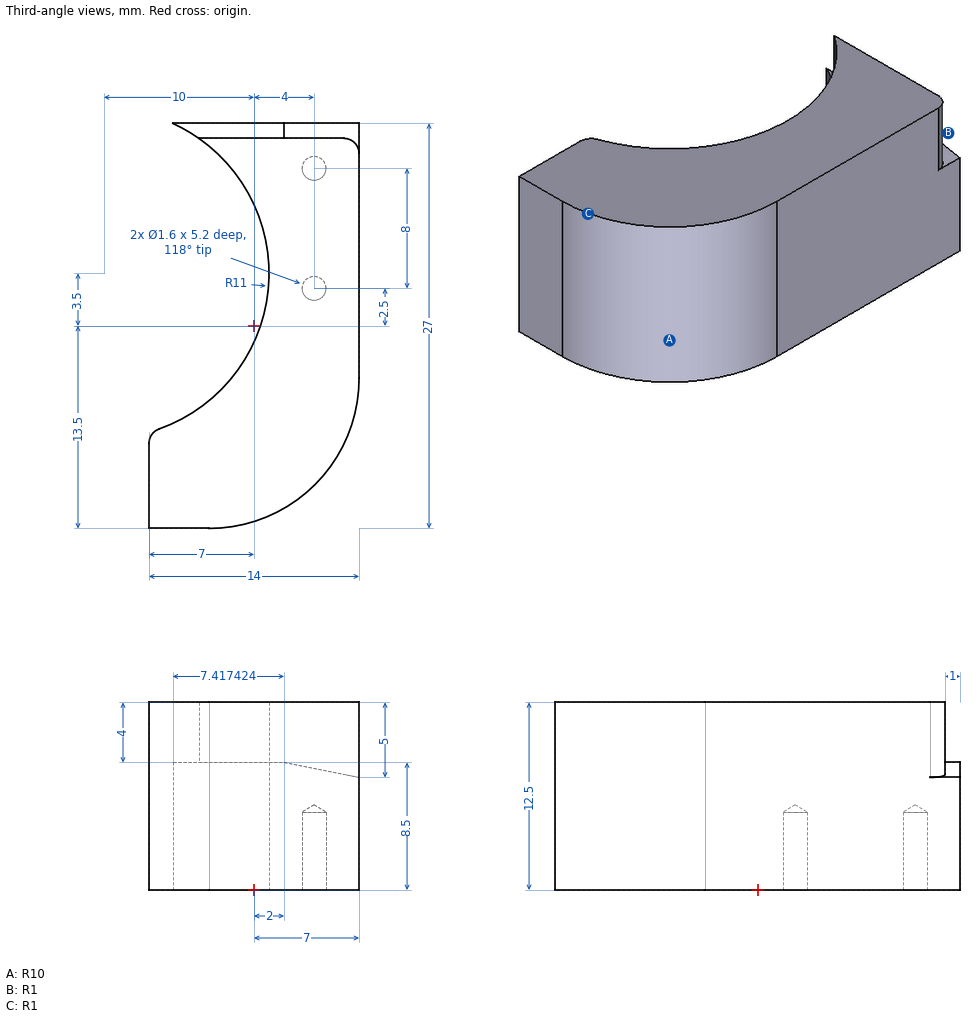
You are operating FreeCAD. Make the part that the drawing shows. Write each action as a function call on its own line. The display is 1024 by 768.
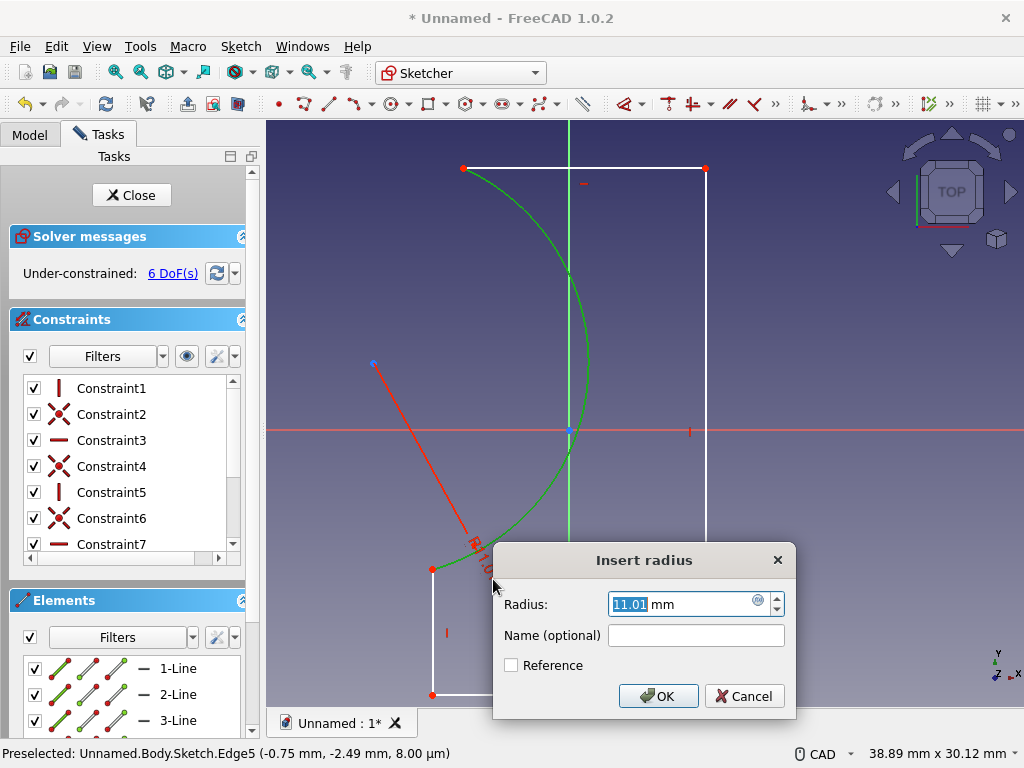
text(11)
key(Return)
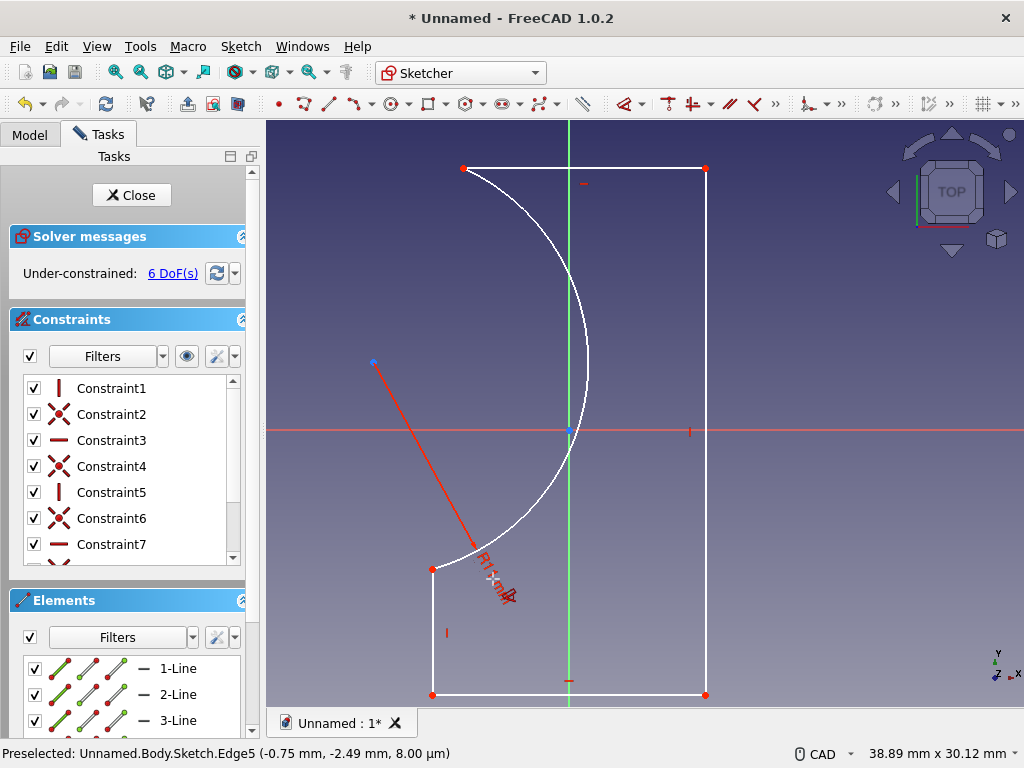
scroll(591, 379, down, 2)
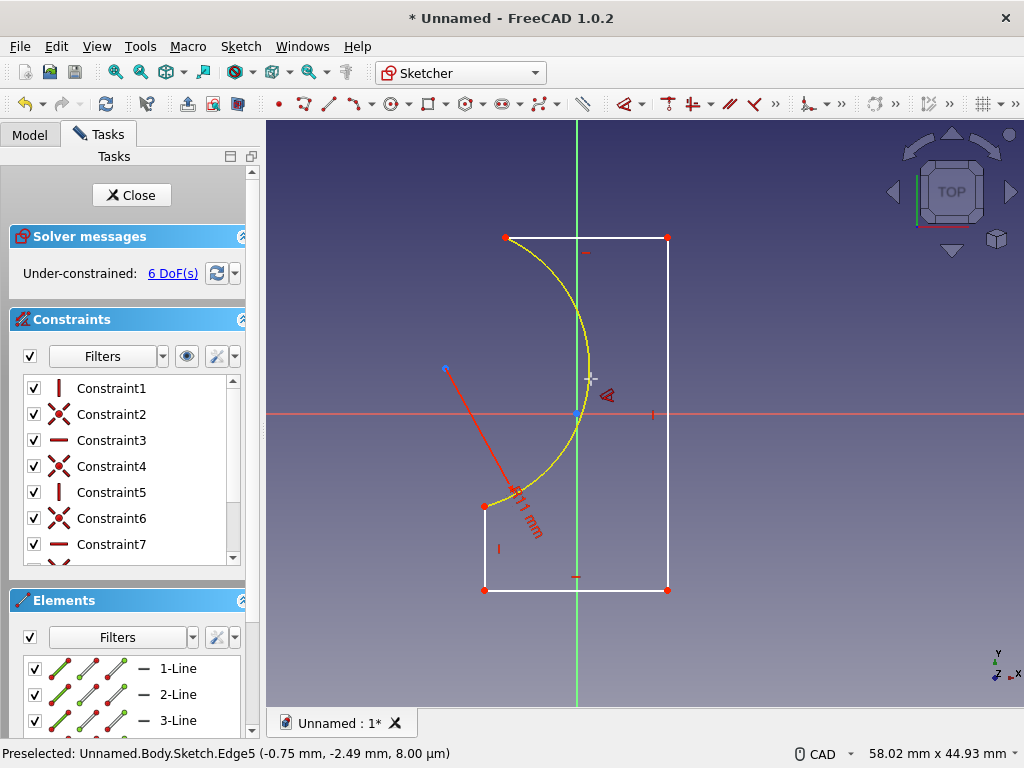
click(540, 591)
click(534, 625)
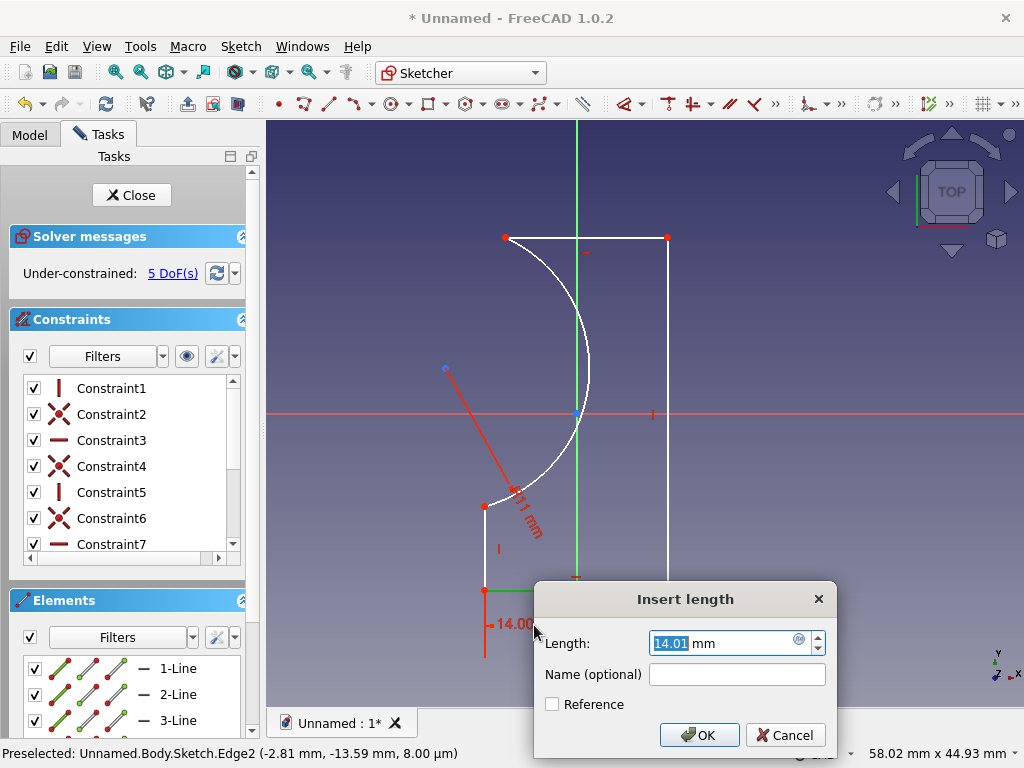
text(14)
key(Return)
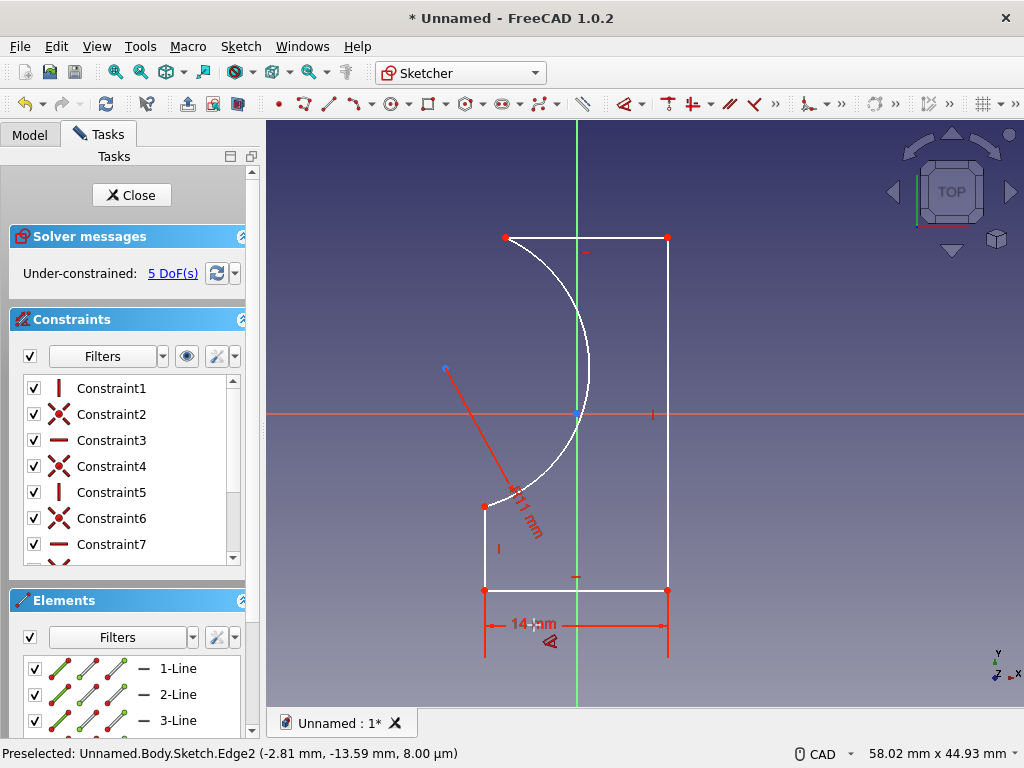
click(668, 485)
click(702, 333)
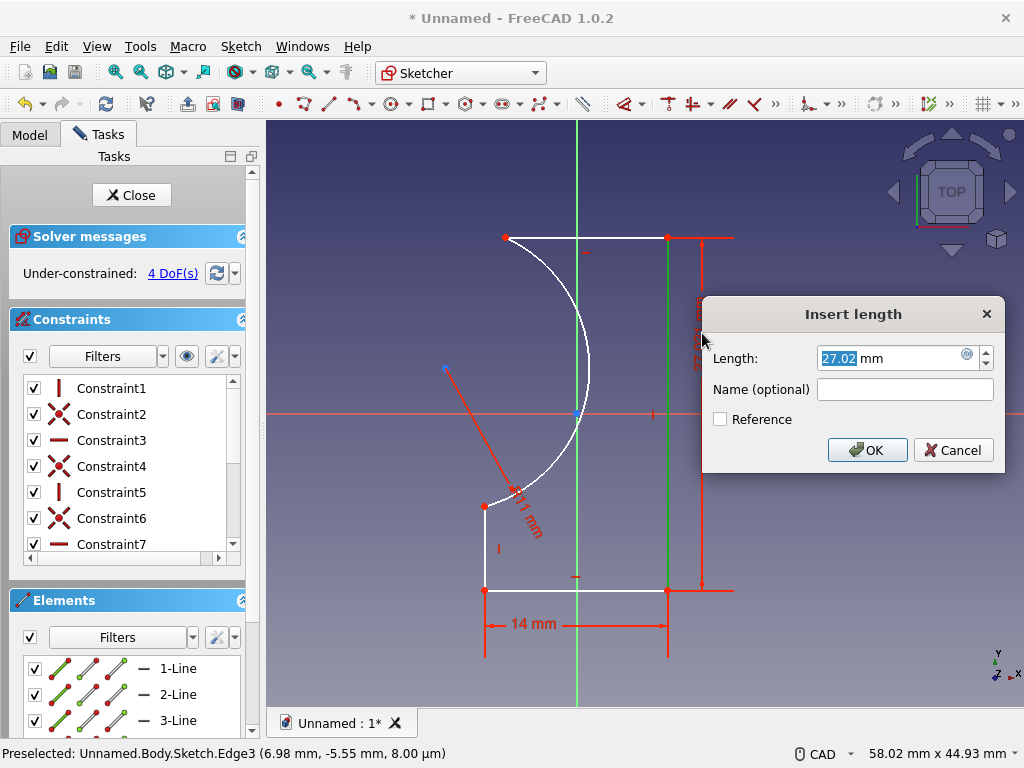
text(27)
key(Return)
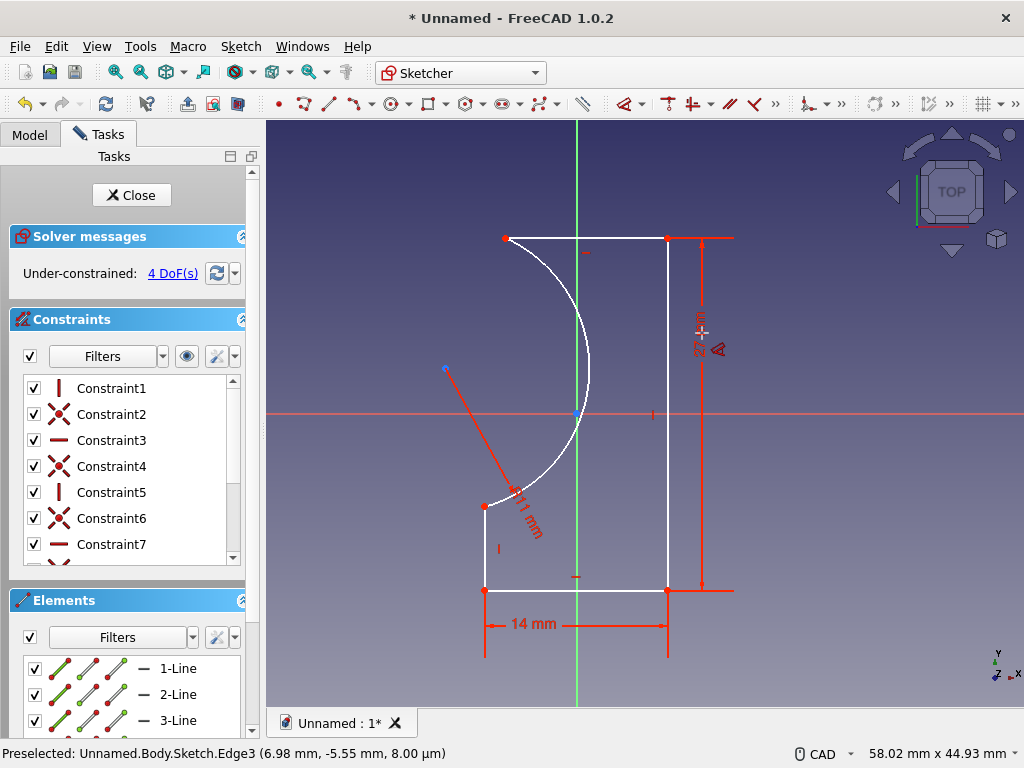
click(485, 507)
click(531, 541)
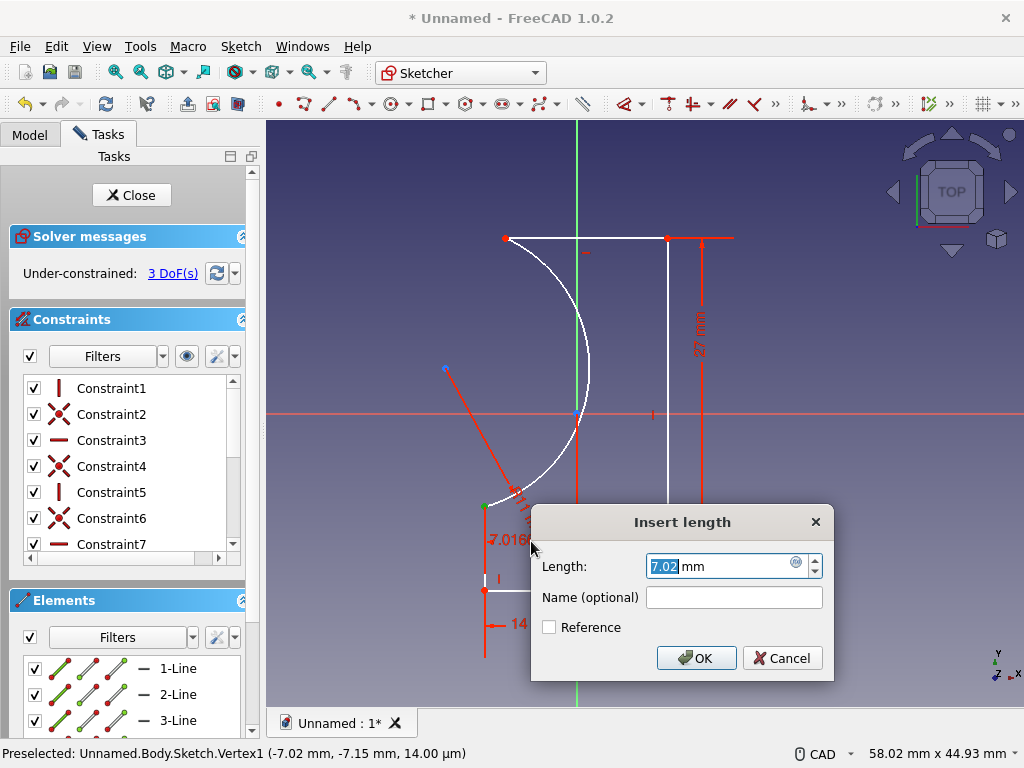
text(7)
key(Return)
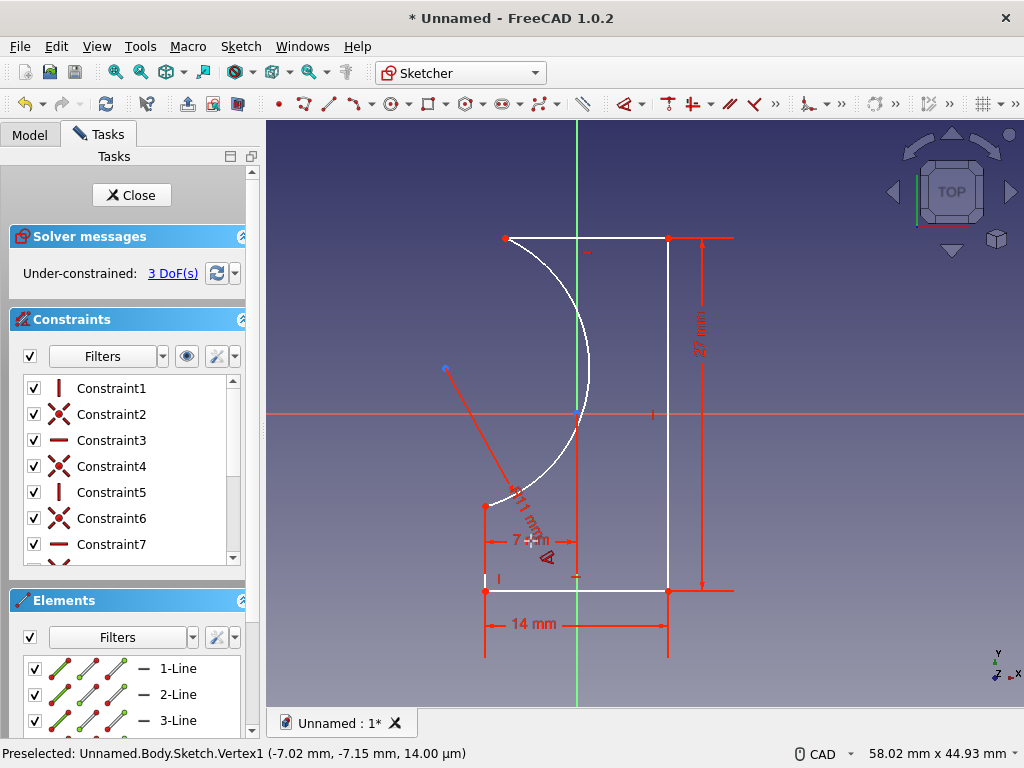
click(446, 369)
click(511, 335)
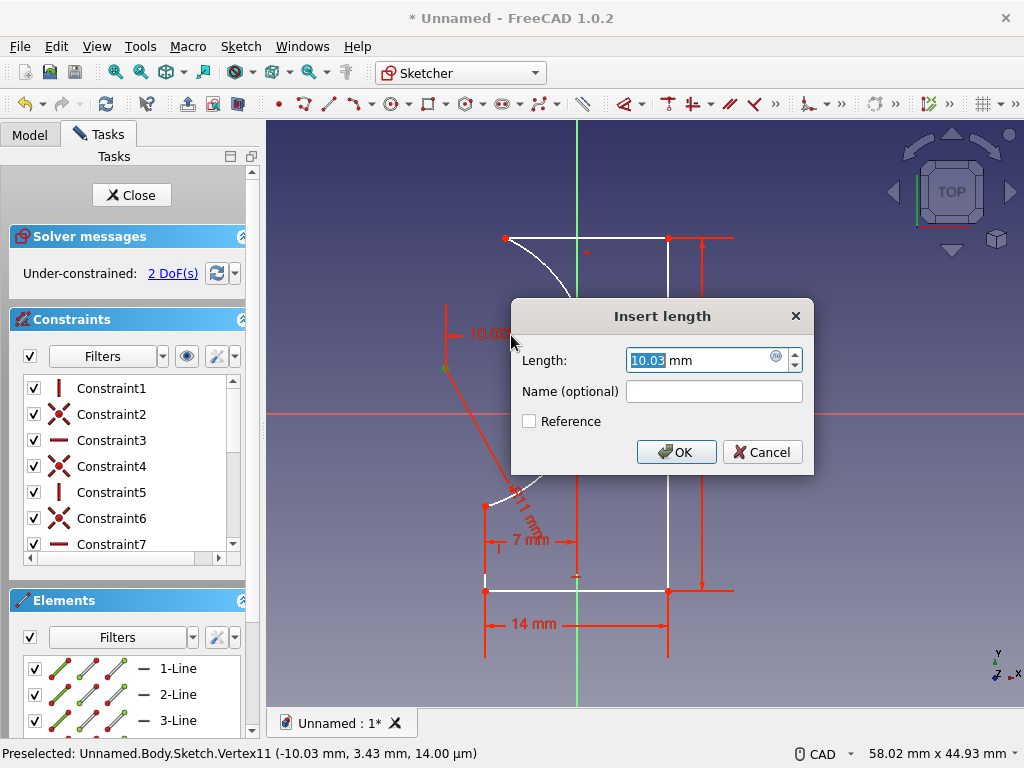
text(10)
key(Return)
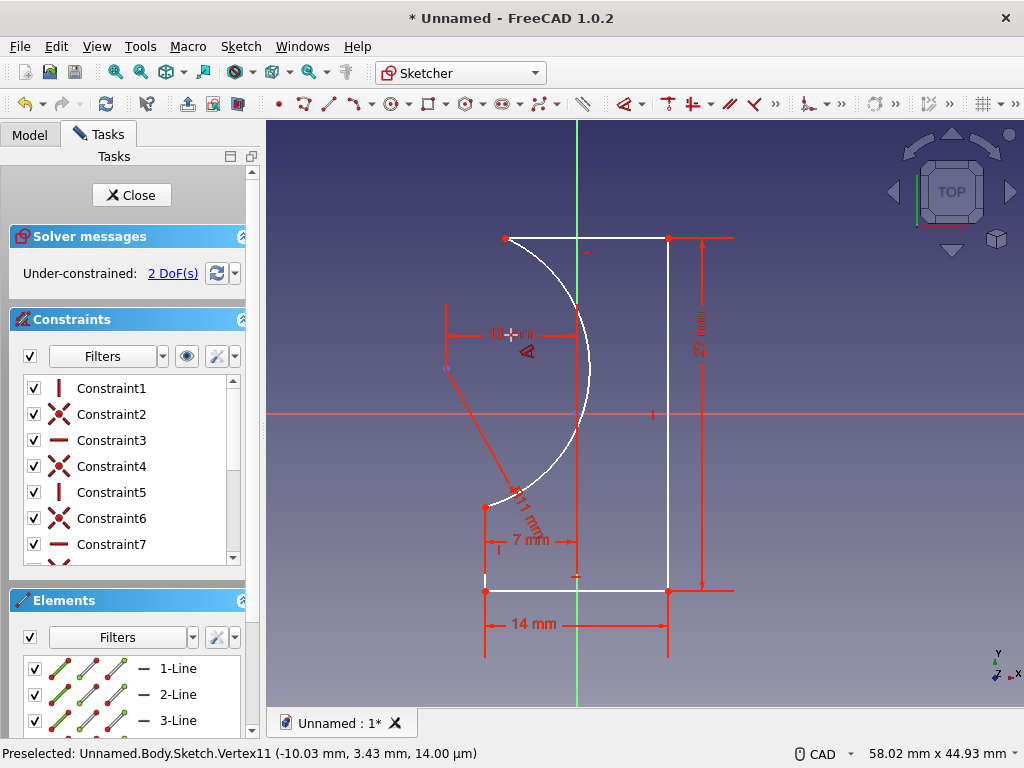
click(446, 369)
click(412, 391)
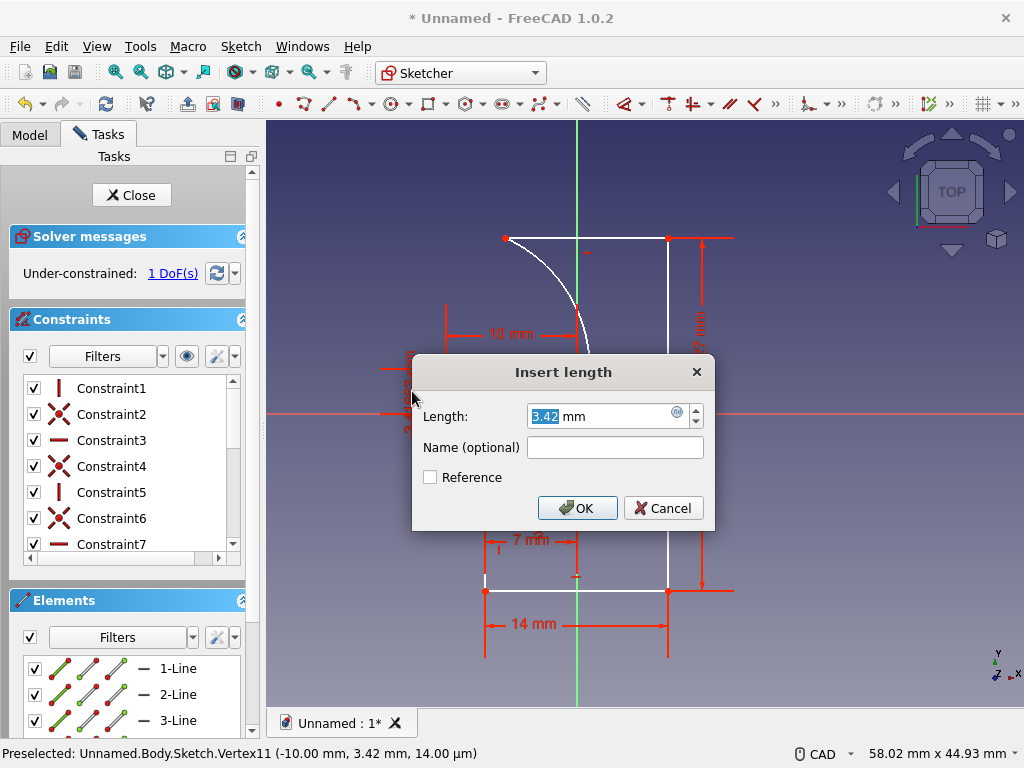
text(3.5)
key(Return)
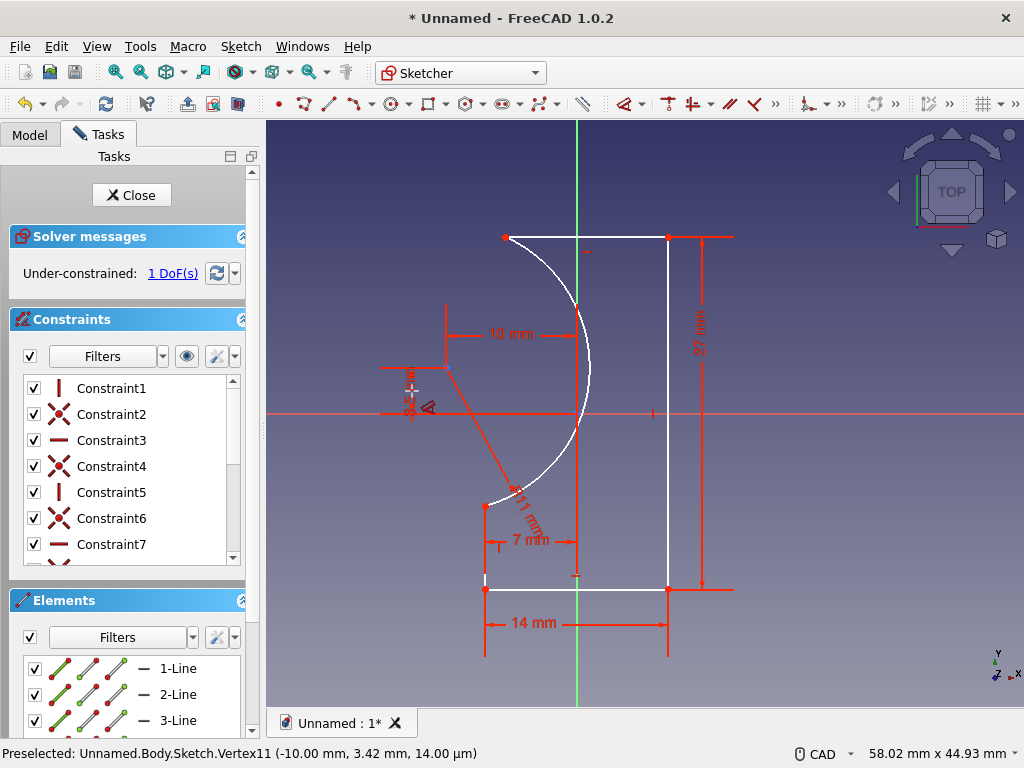
click(485, 590)
click(451, 502)